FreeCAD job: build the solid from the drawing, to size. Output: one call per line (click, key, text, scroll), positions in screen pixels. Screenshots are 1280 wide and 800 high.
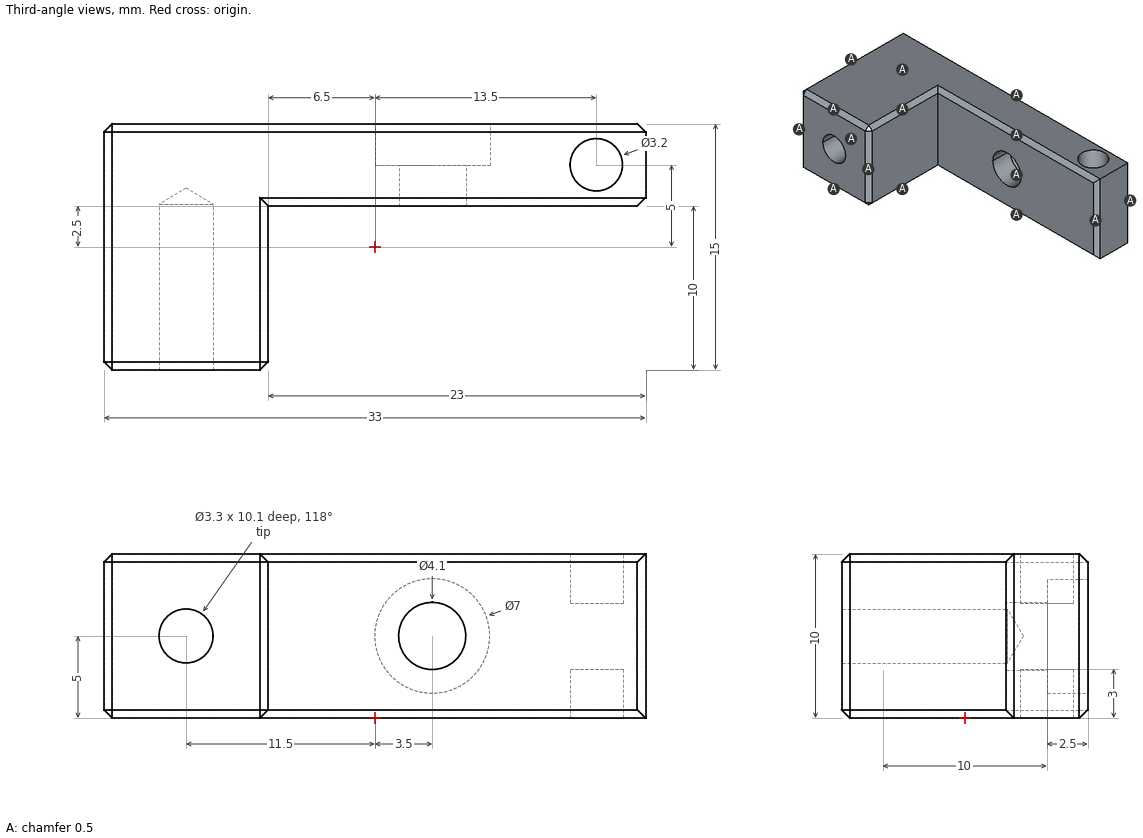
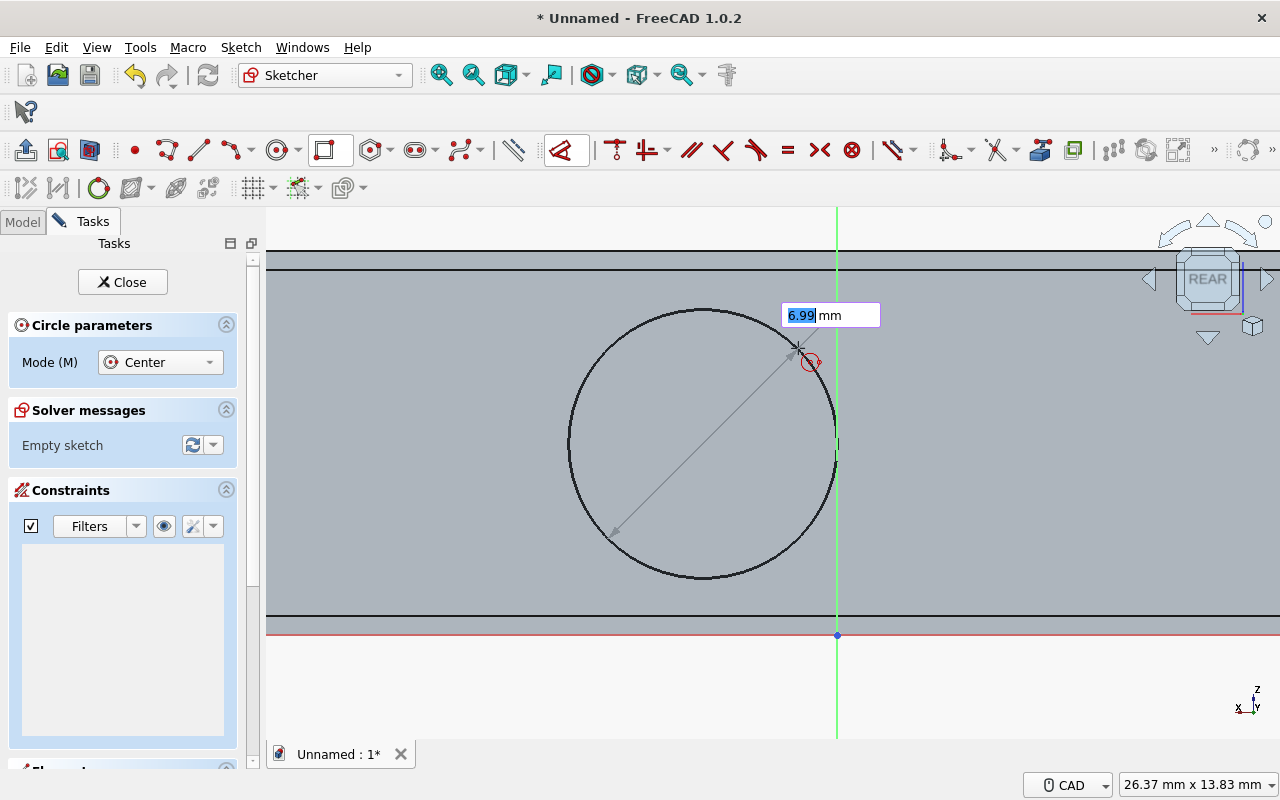
text(7)
key(Return)
key(Escape)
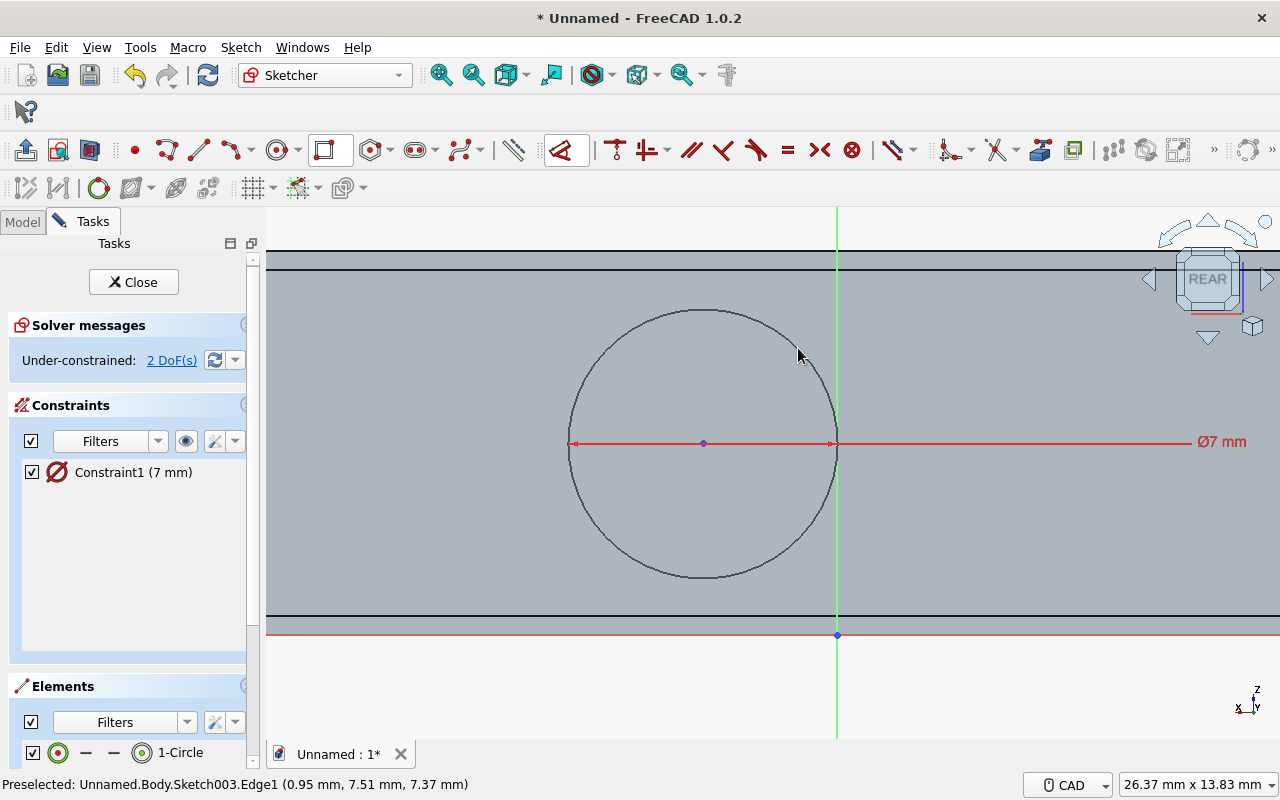
click(703, 444)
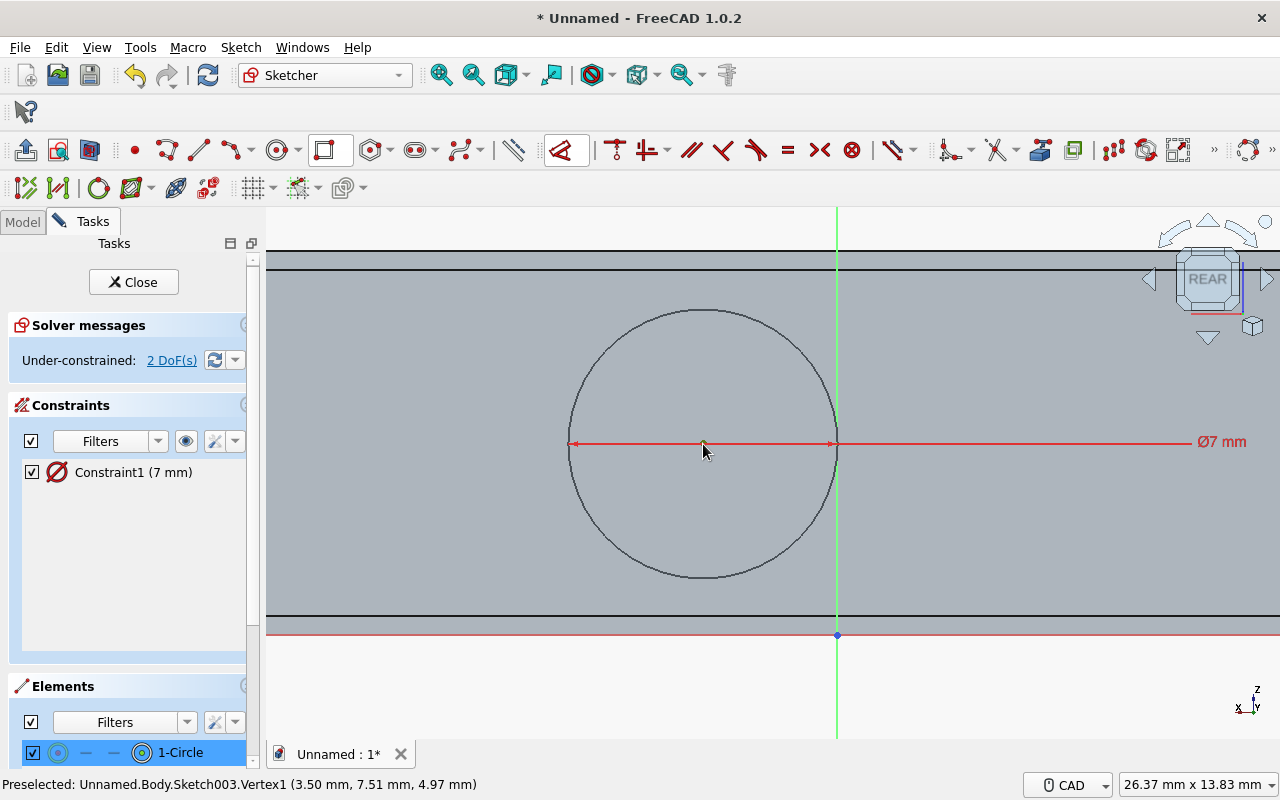
key(i)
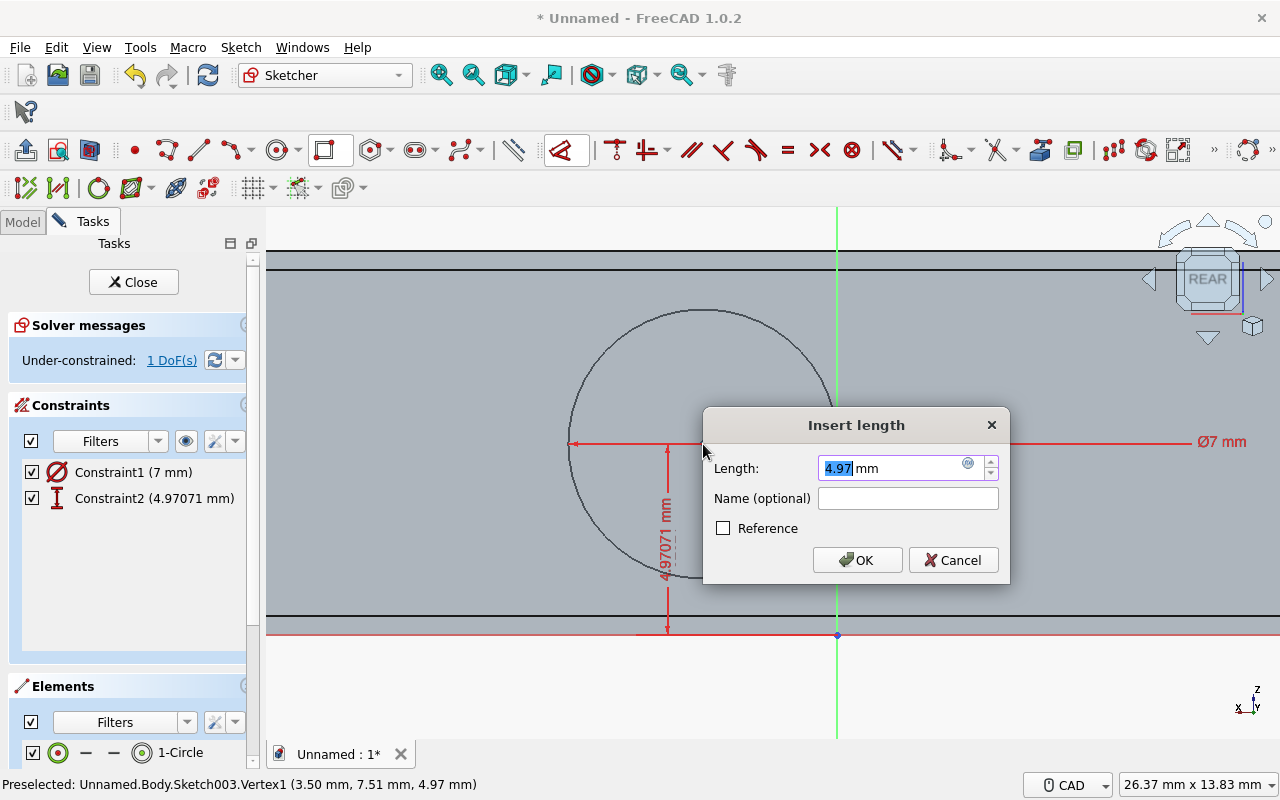
text(5)
key(Return)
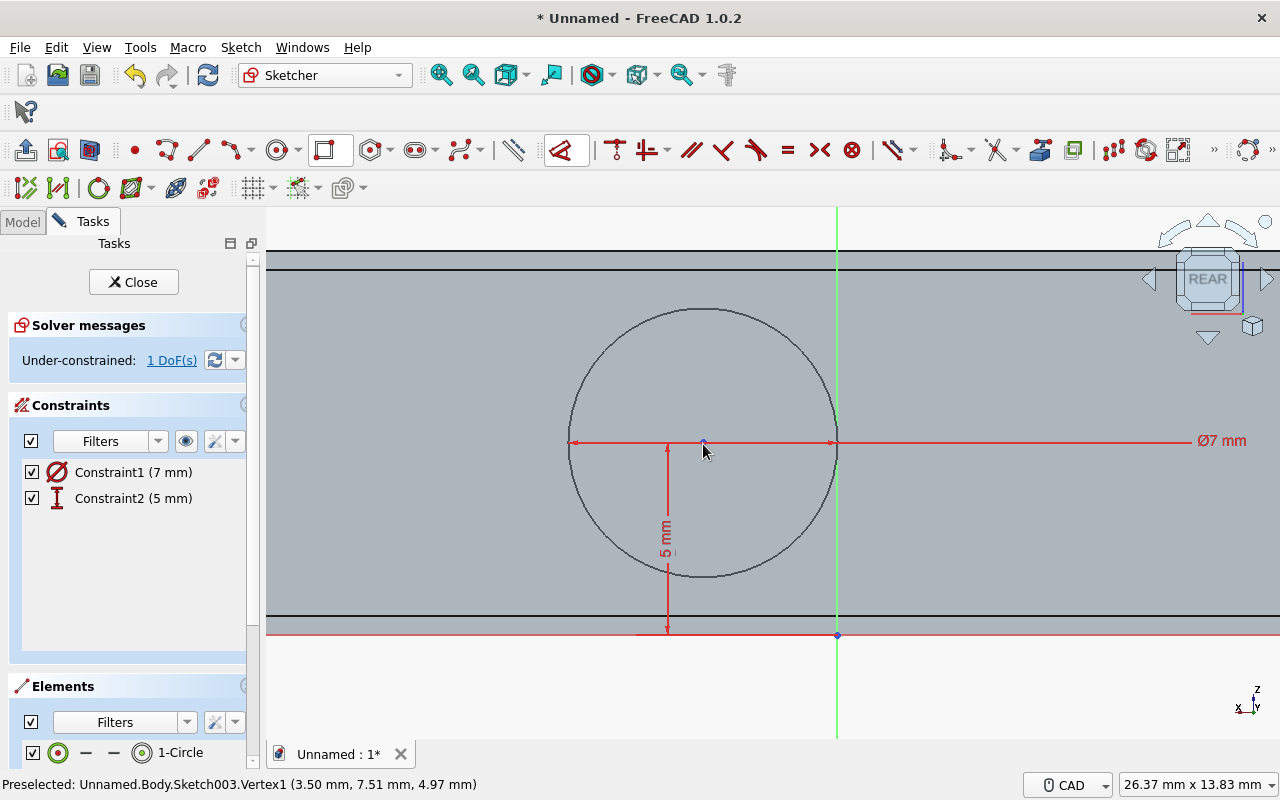
click(703, 443)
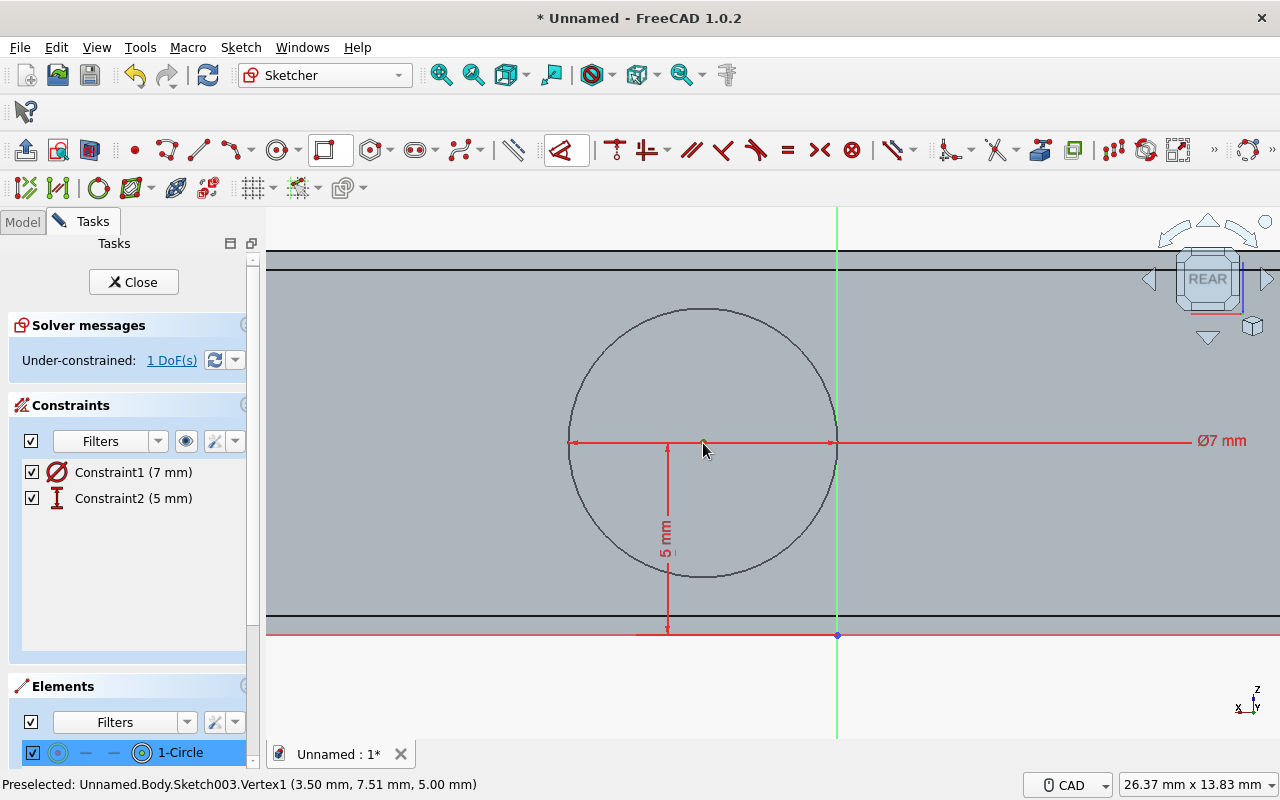
click(584, 150)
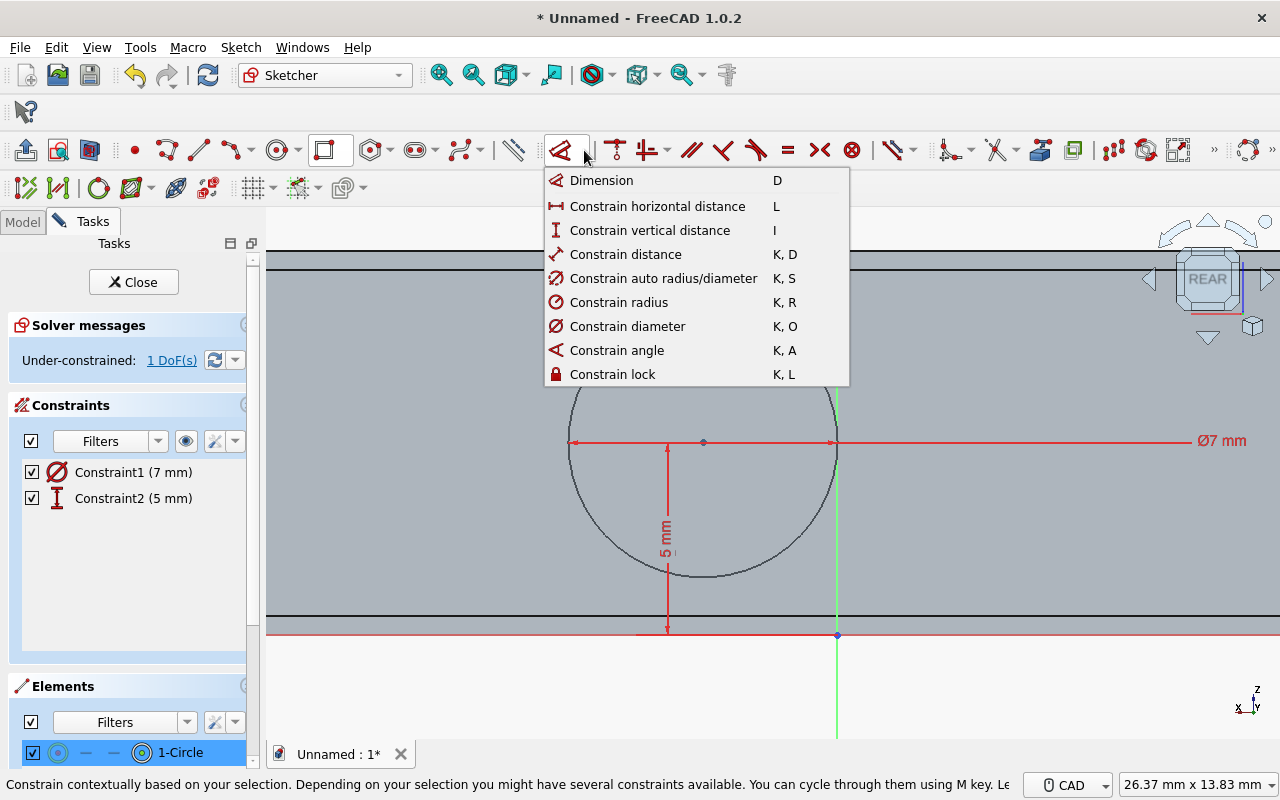
click(697, 206)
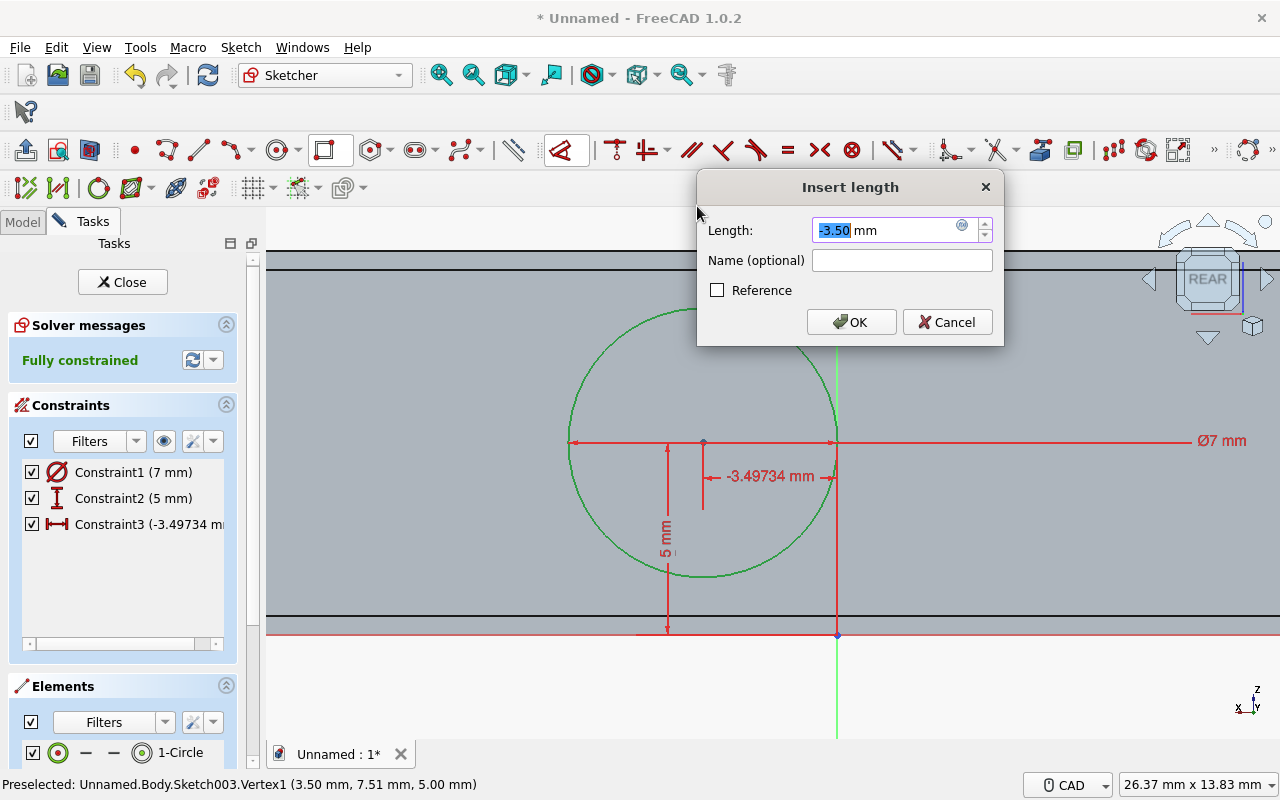
text(-3.5)
key(Return)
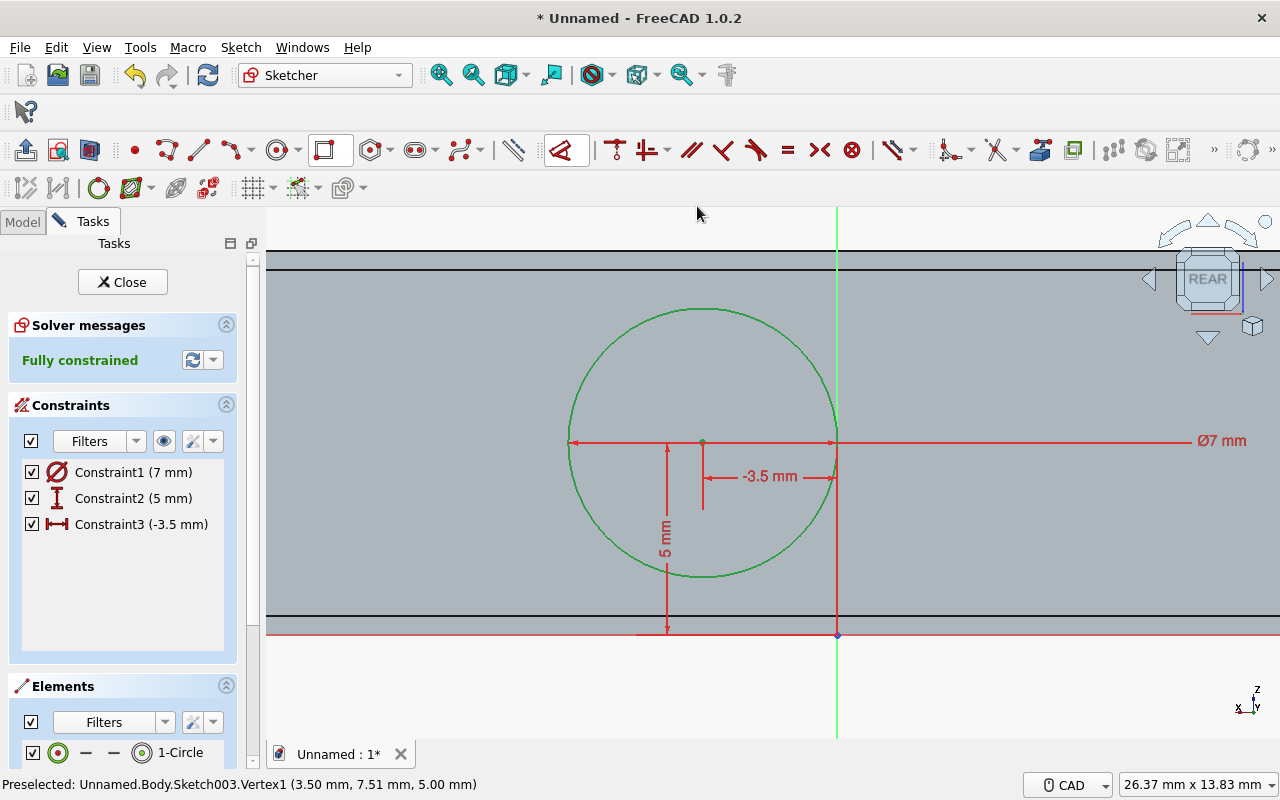
click(123, 282)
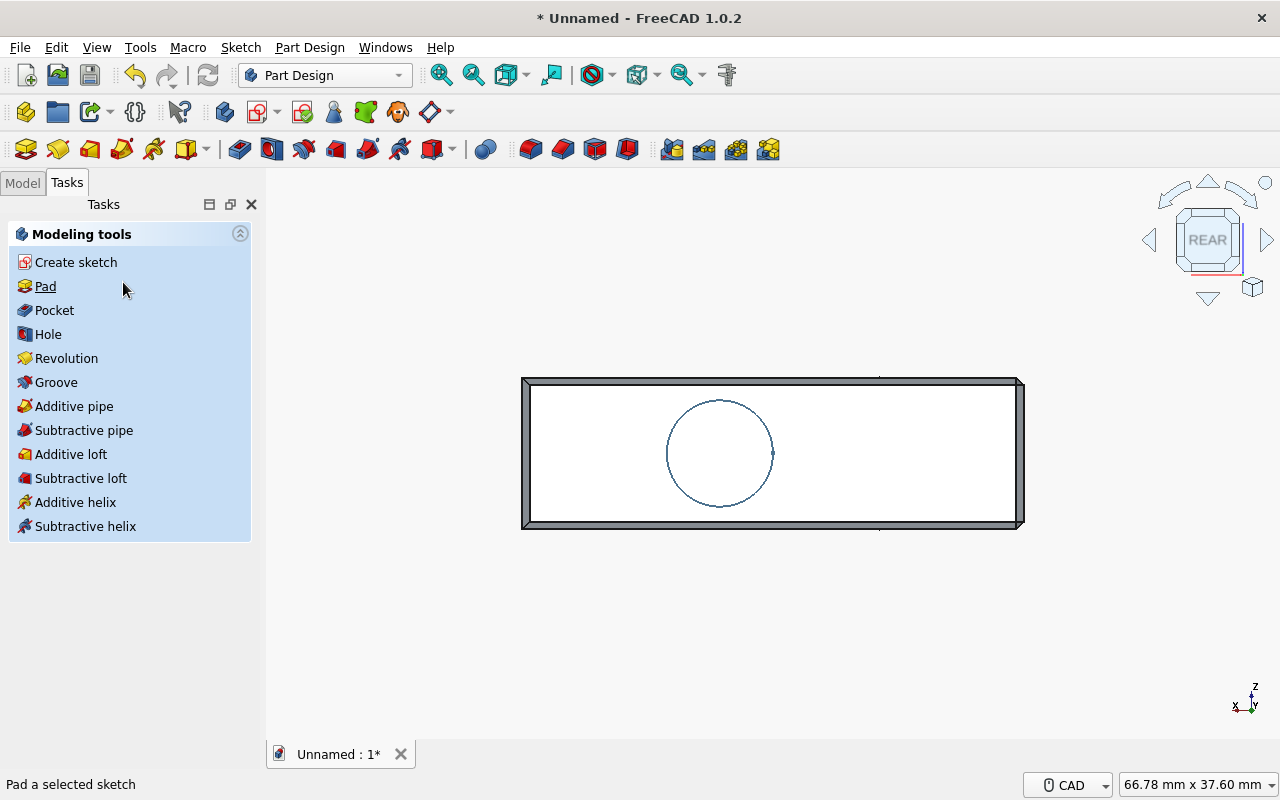
click(240, 150)